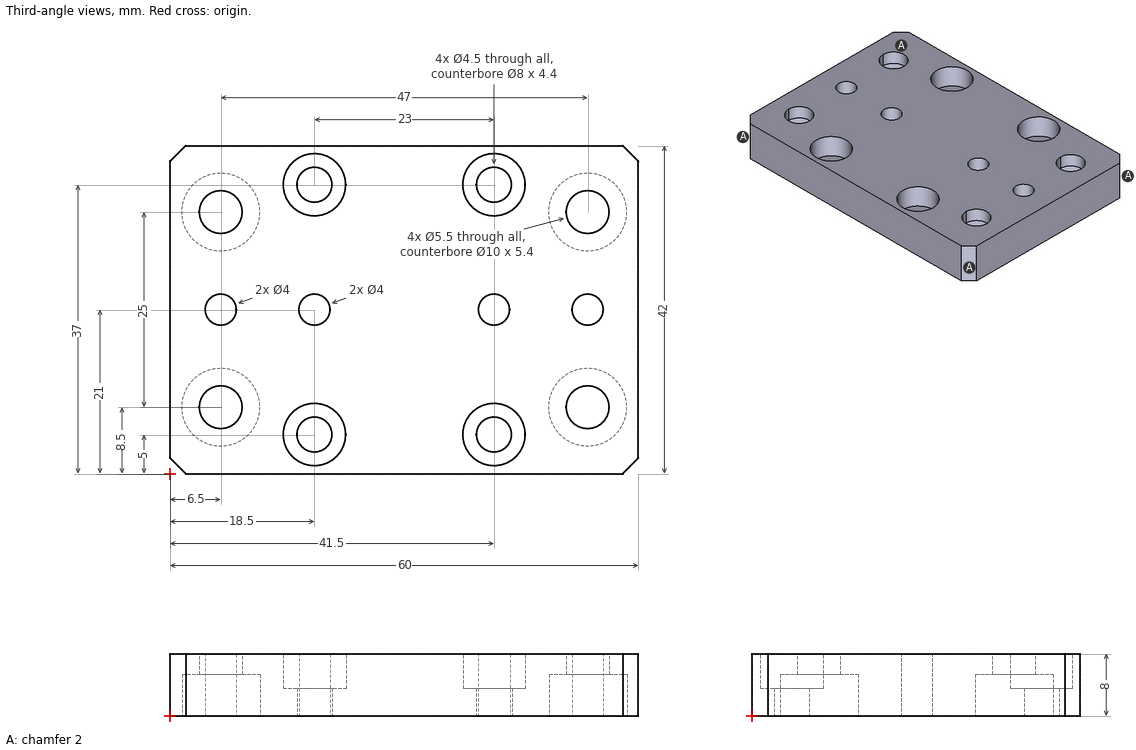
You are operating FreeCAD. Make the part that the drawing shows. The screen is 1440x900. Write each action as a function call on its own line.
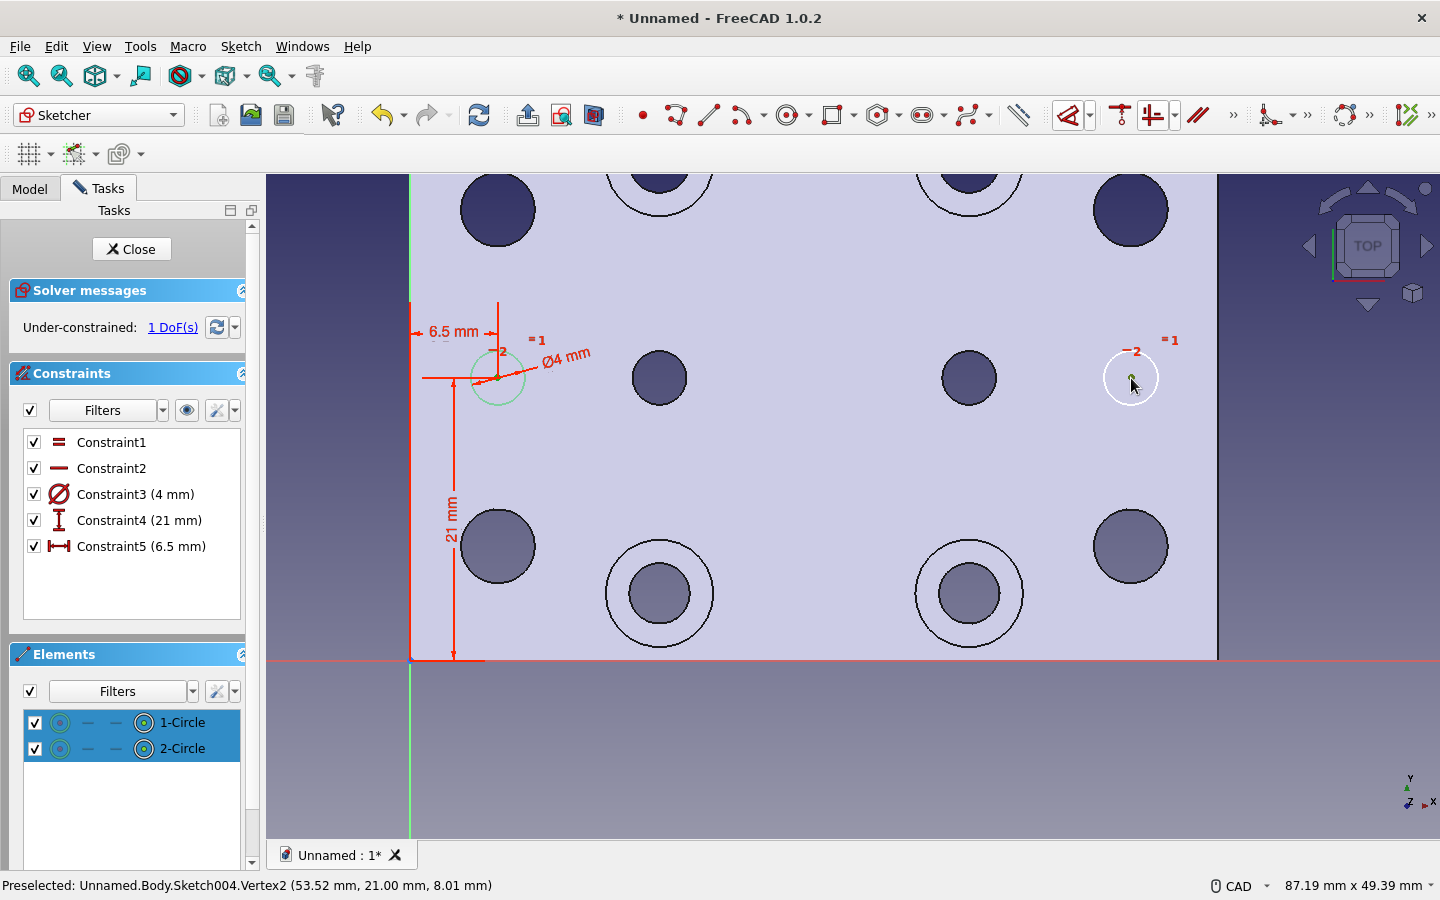
key(l)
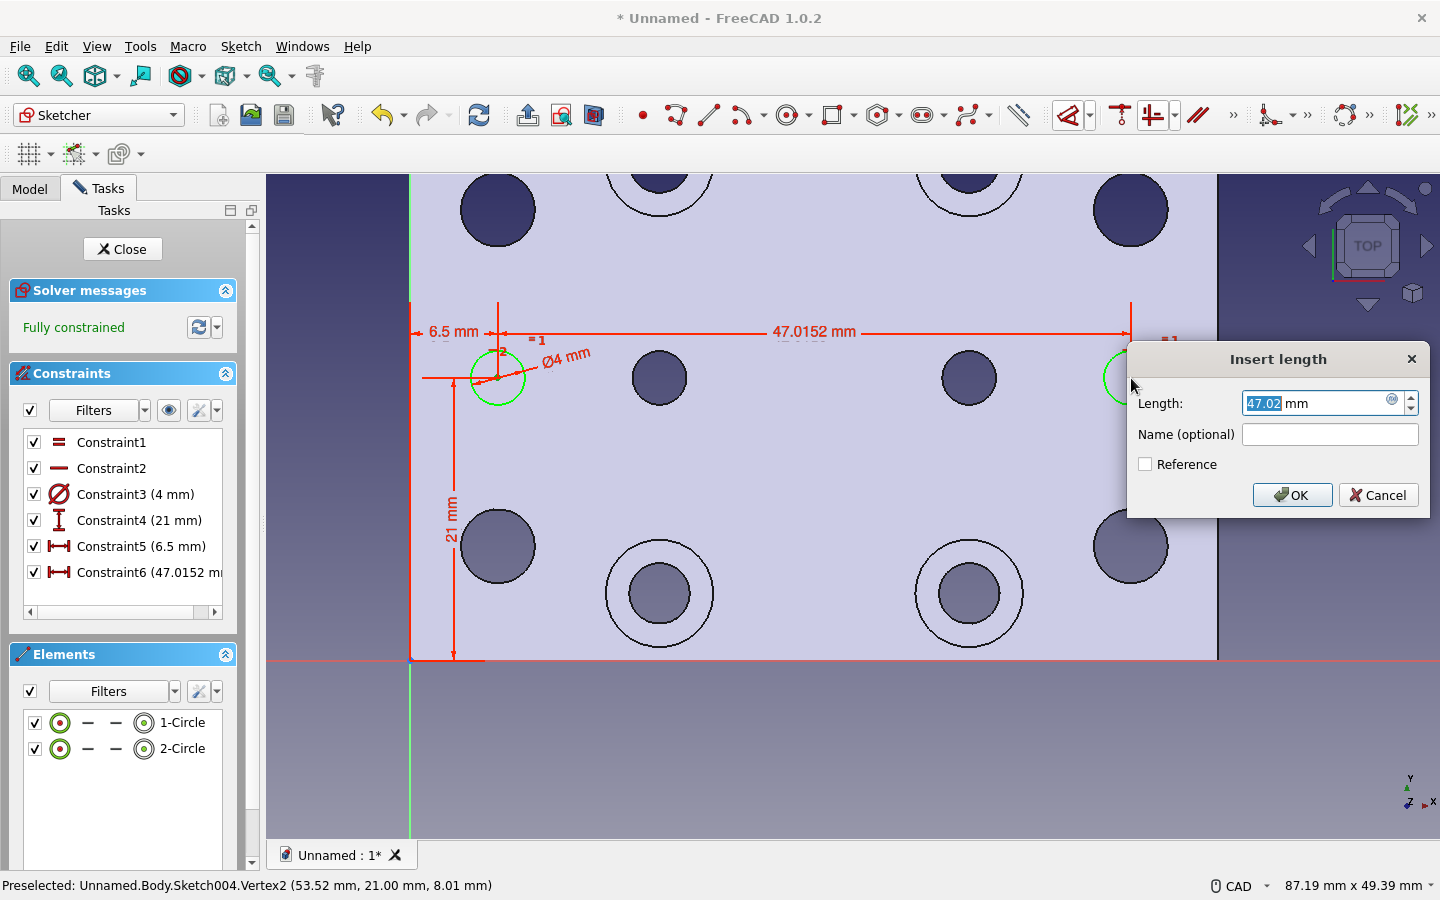
text(47)
key(Return)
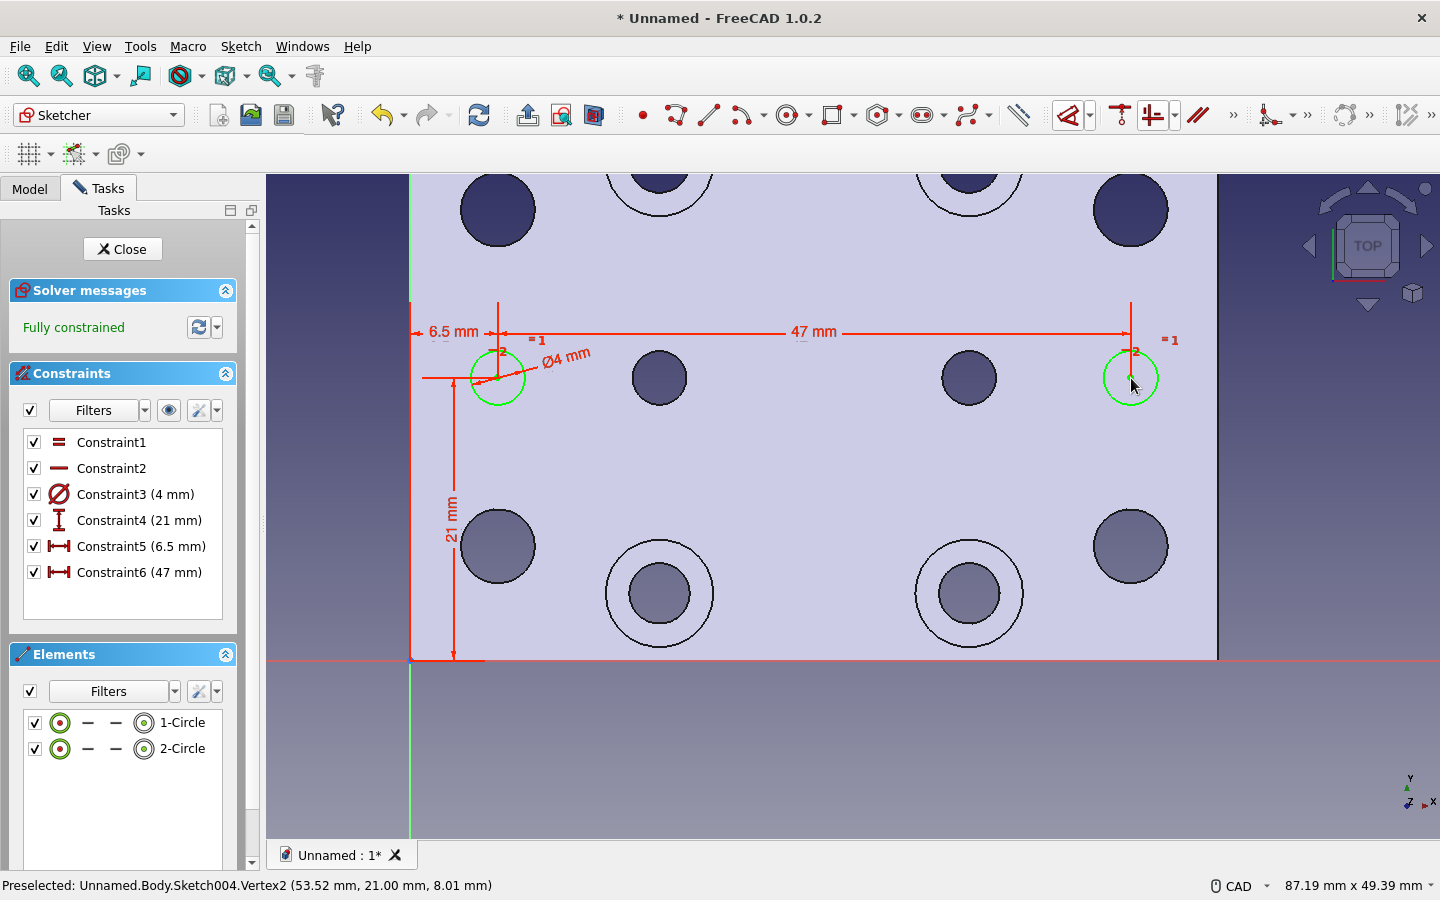
click(123, 249)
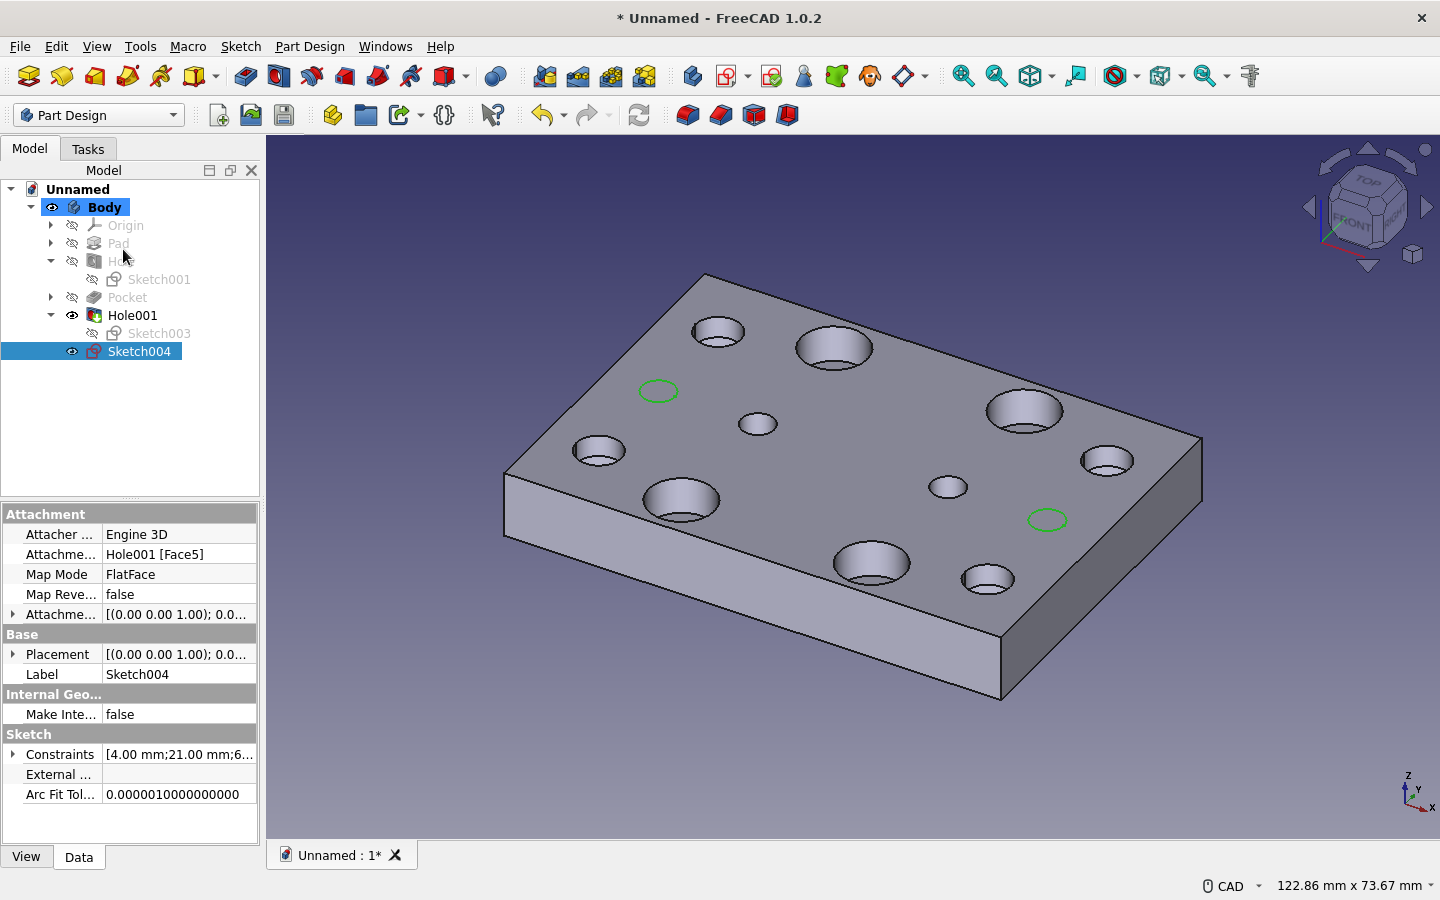
click(246, 76)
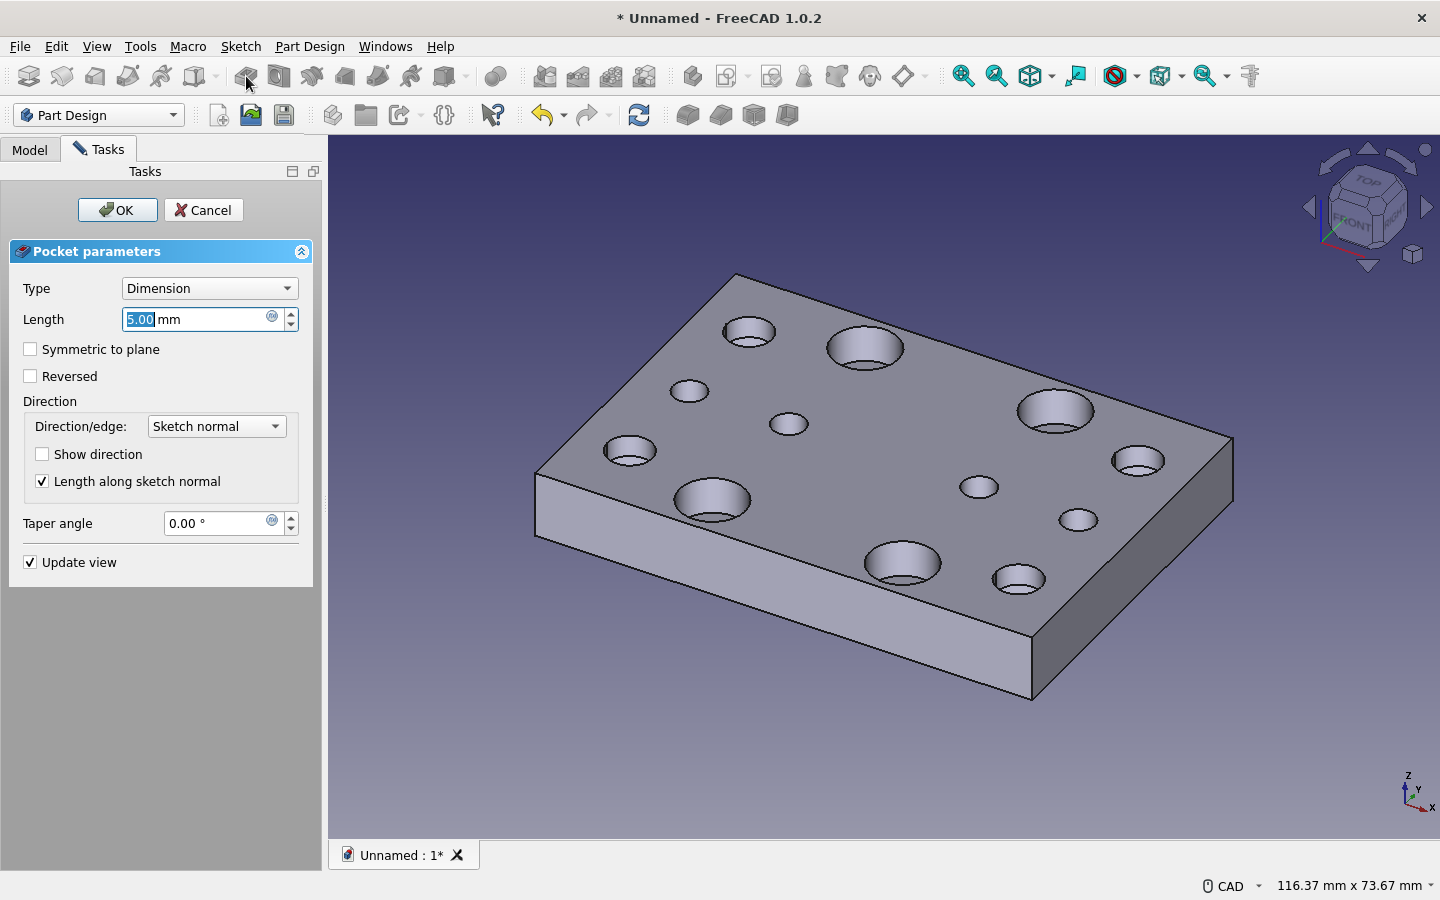
click(210, 288)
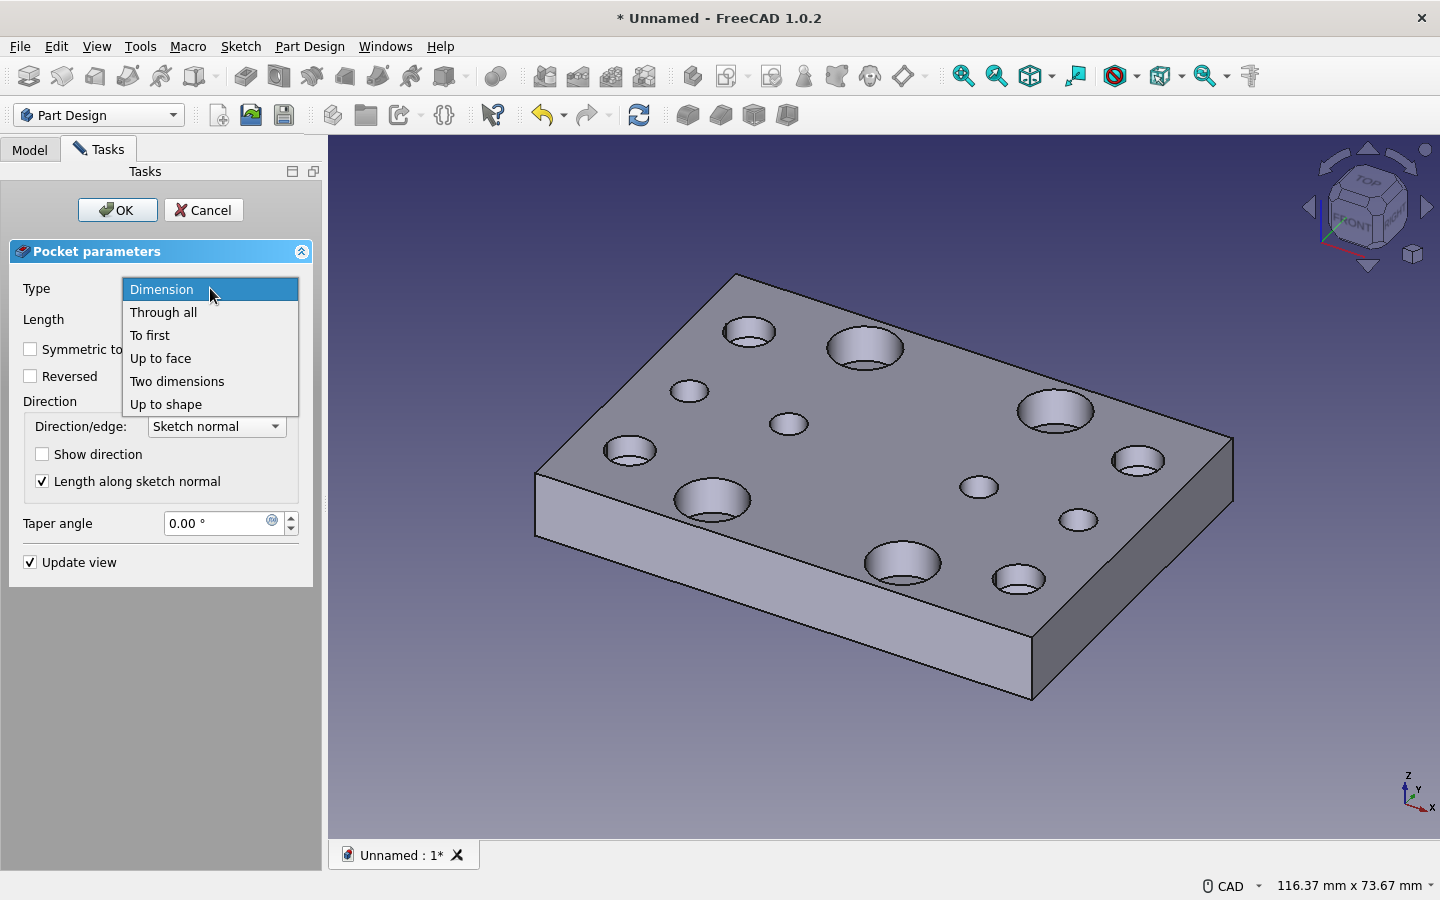
click(208, 312)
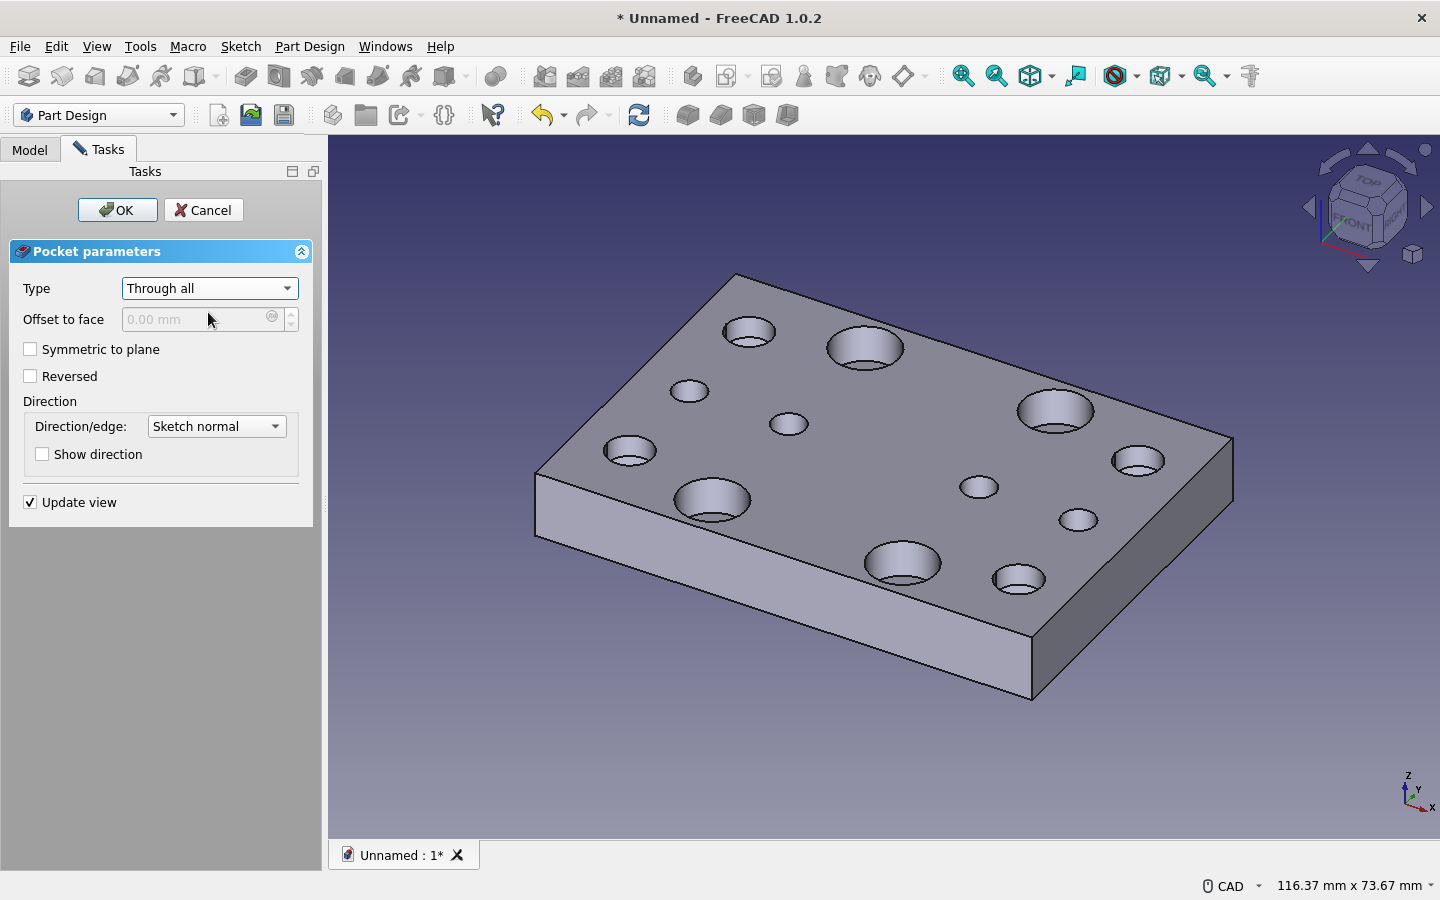
click(118, 210)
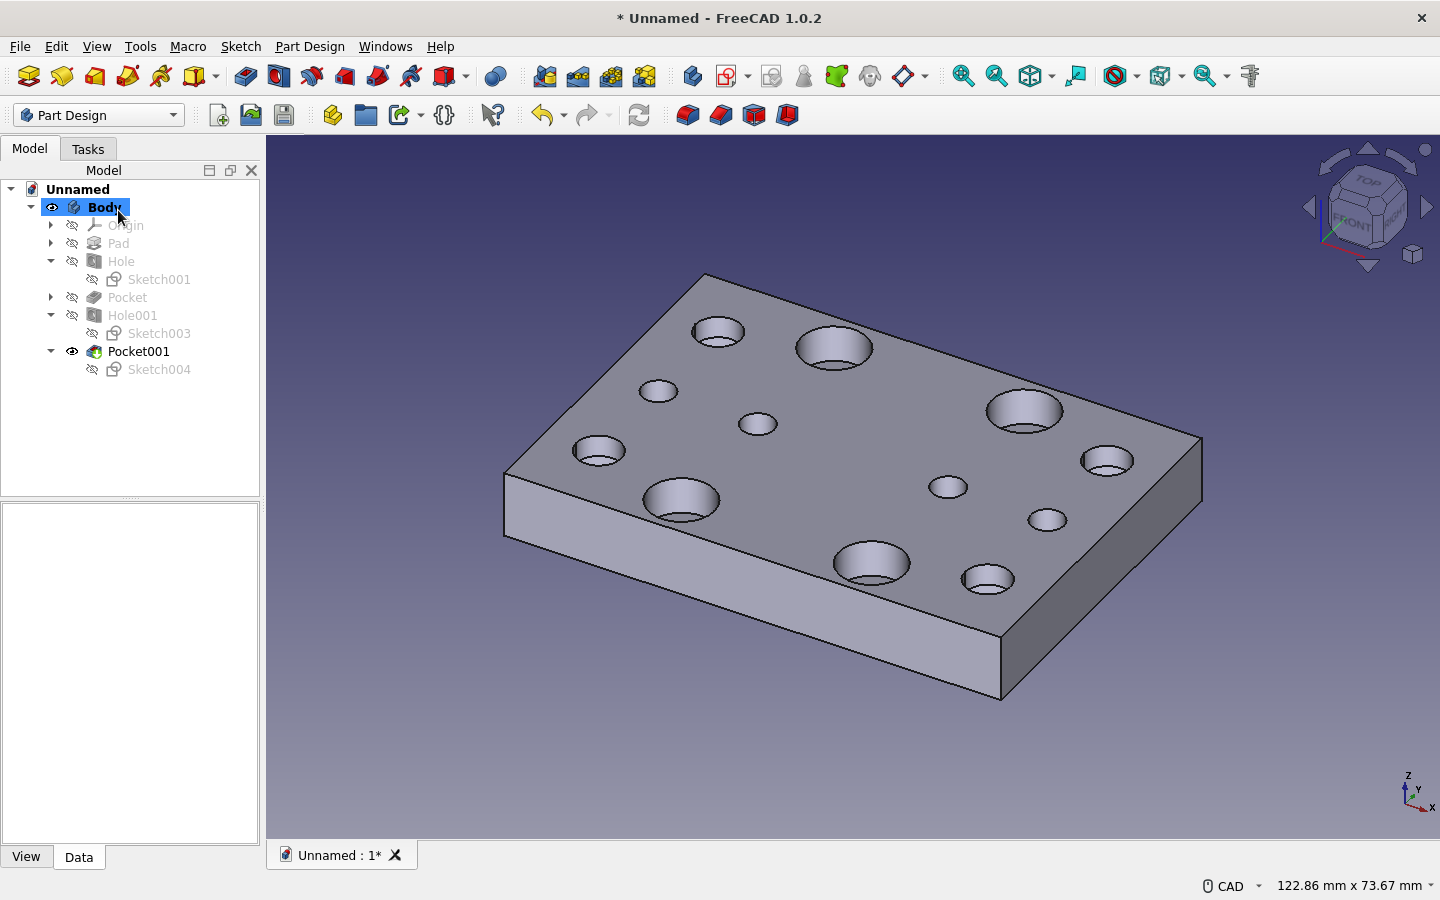
click(1001, 668)